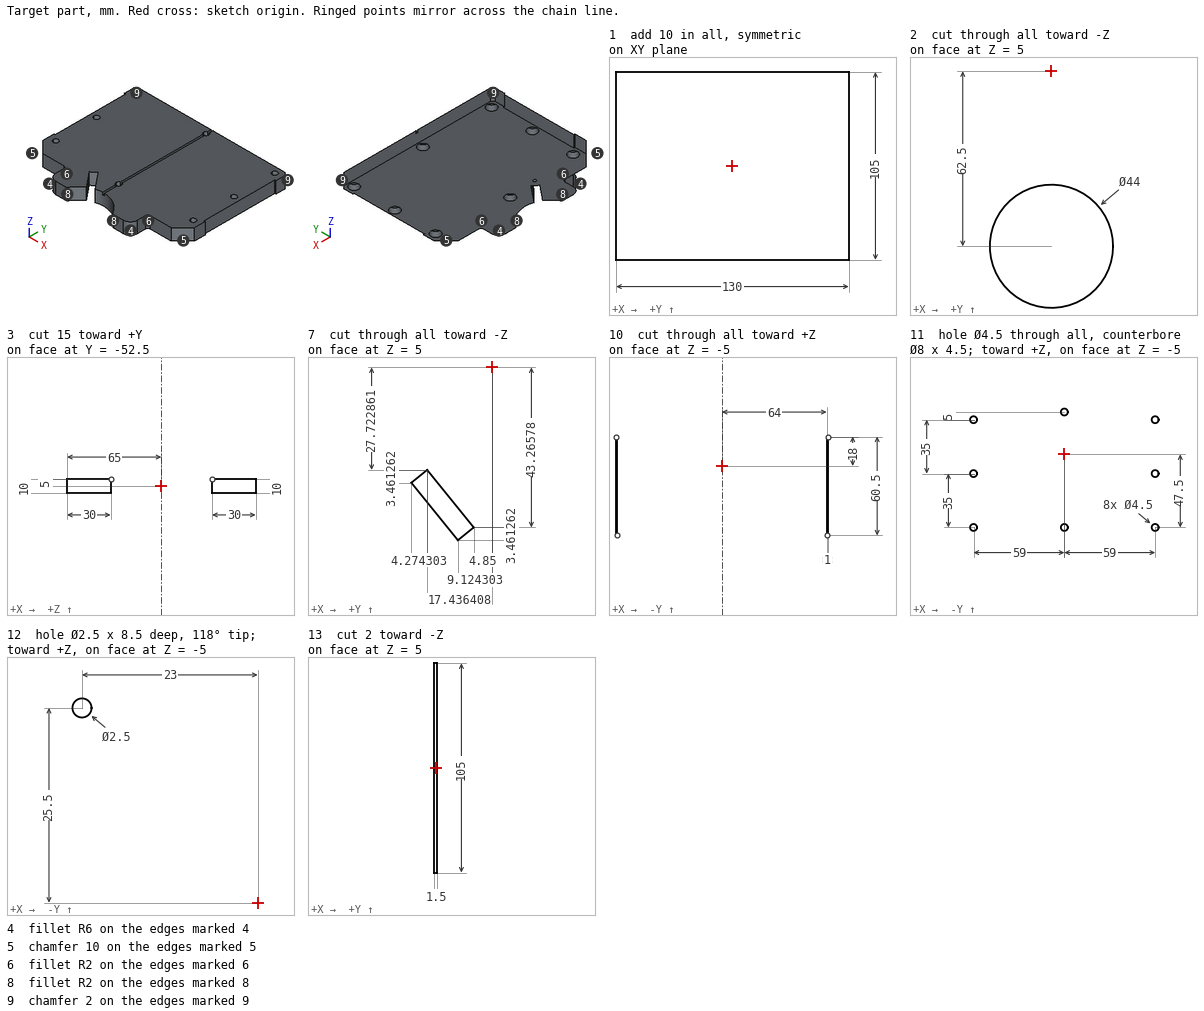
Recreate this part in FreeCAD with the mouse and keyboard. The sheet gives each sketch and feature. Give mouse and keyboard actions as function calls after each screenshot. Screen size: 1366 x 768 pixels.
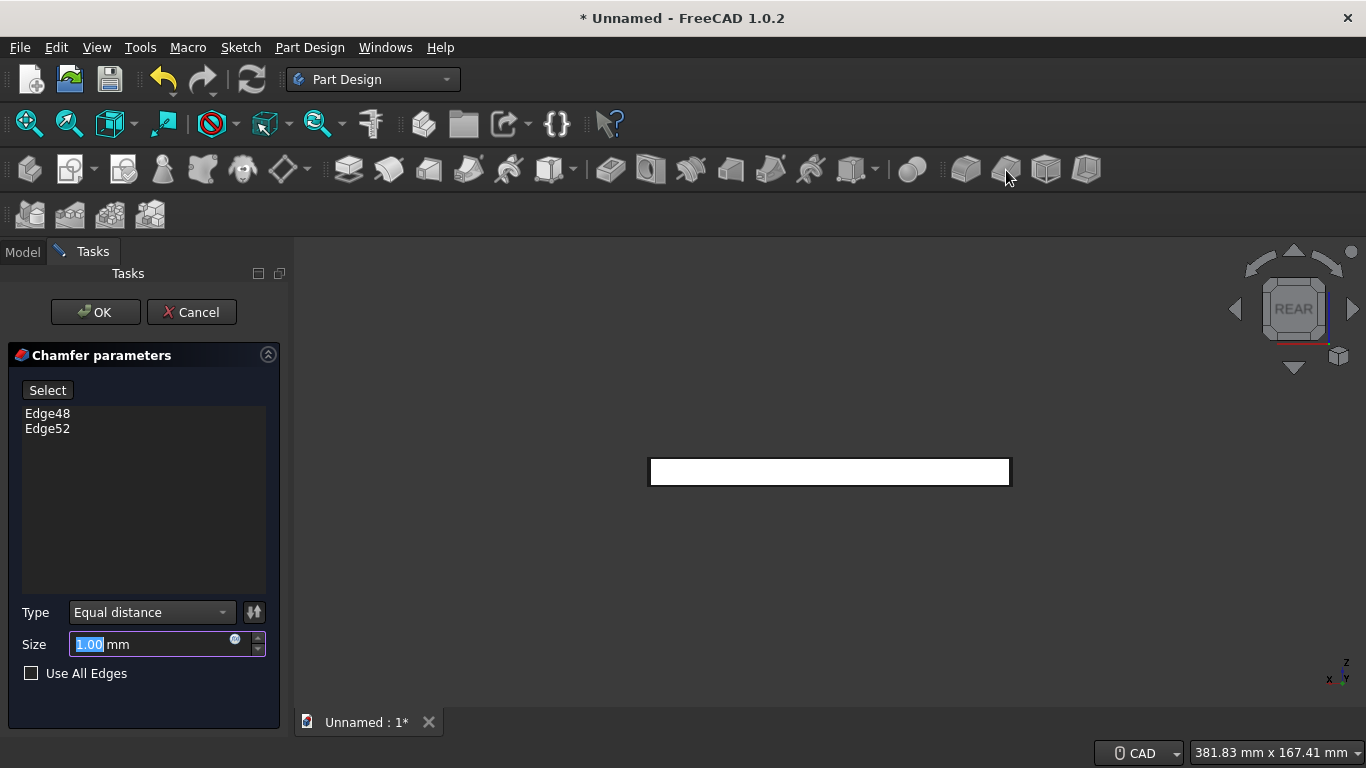
text(2)
key(Tab)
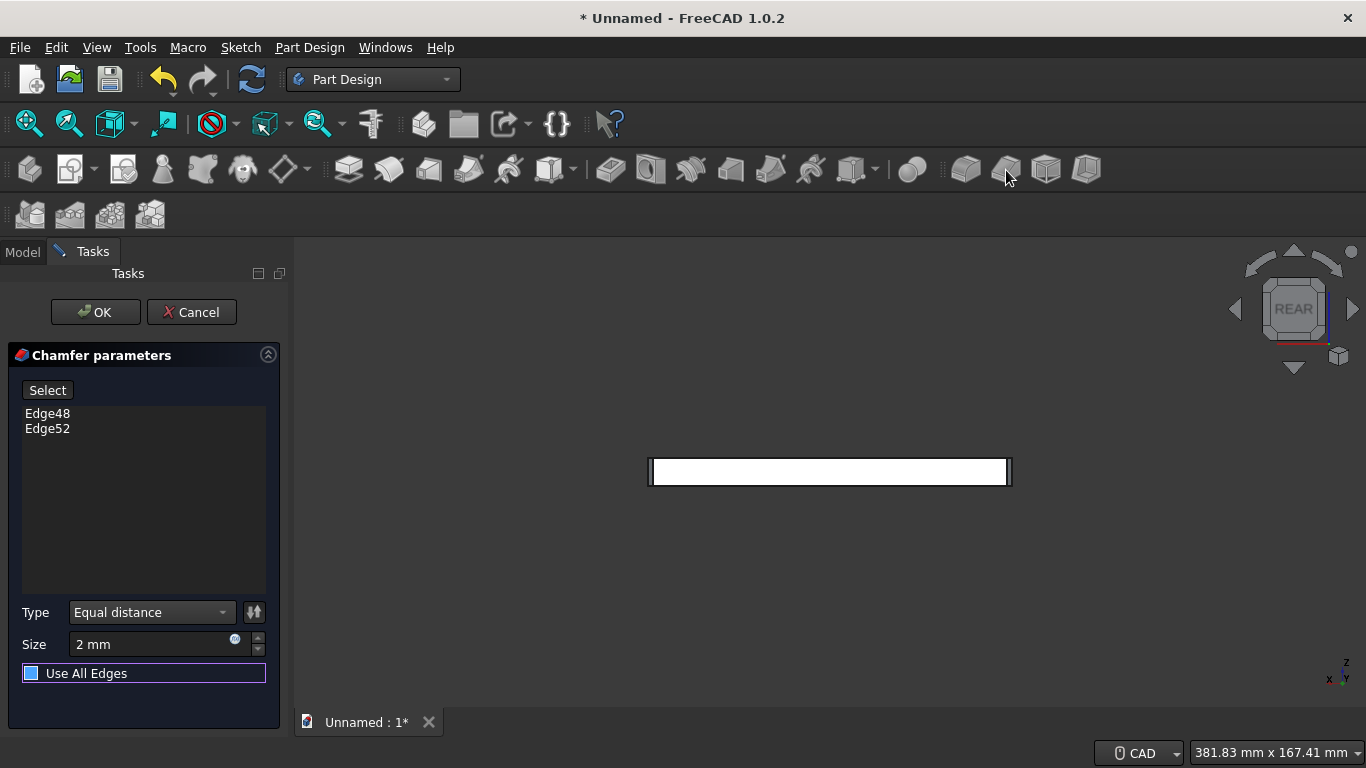
click(96, 312)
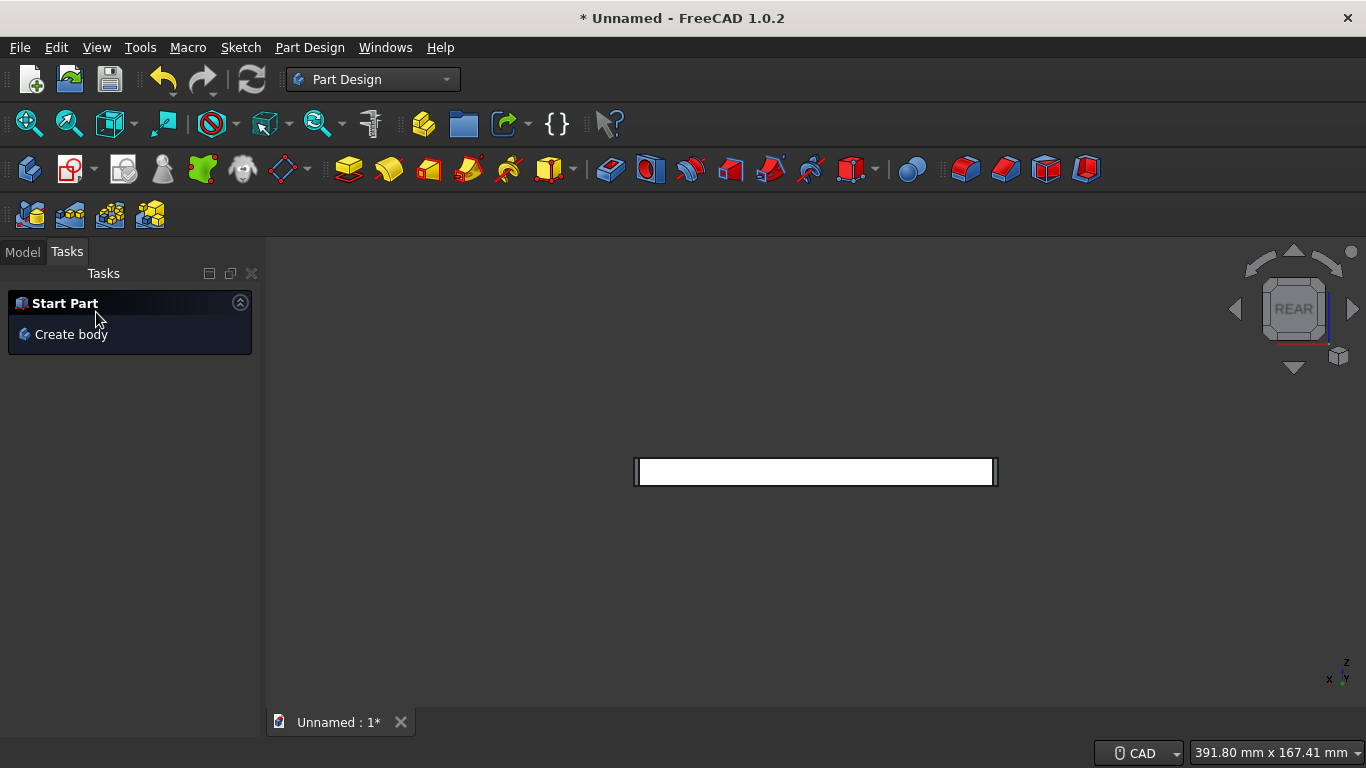
click(30, 124)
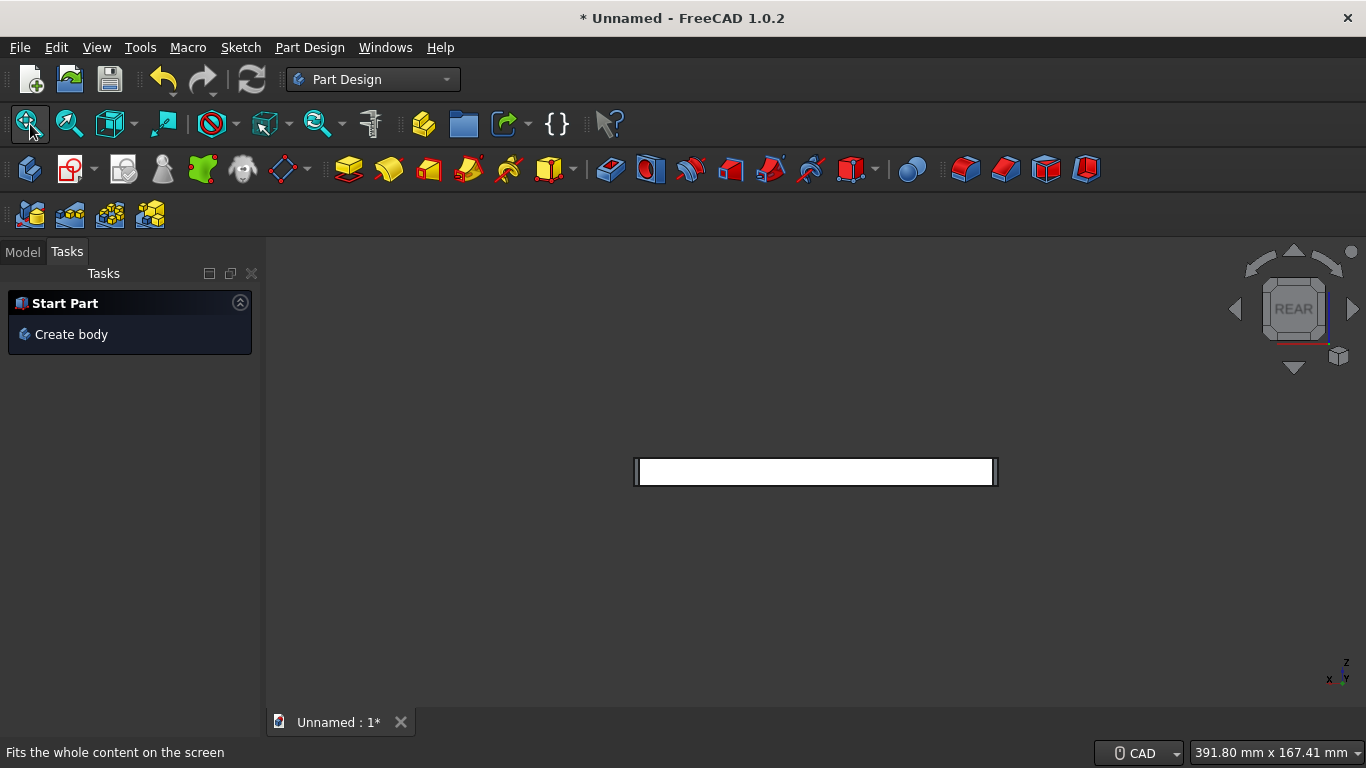
key(5)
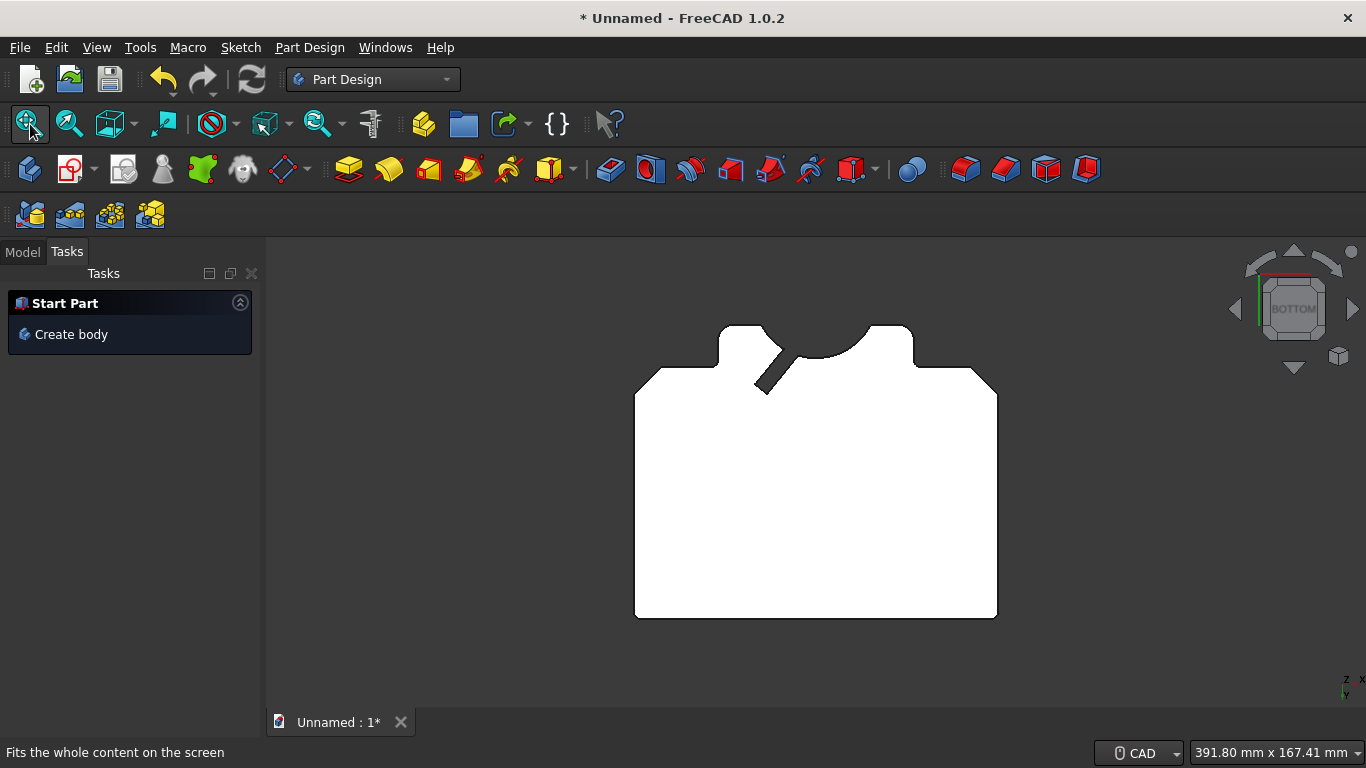
click(868, 471)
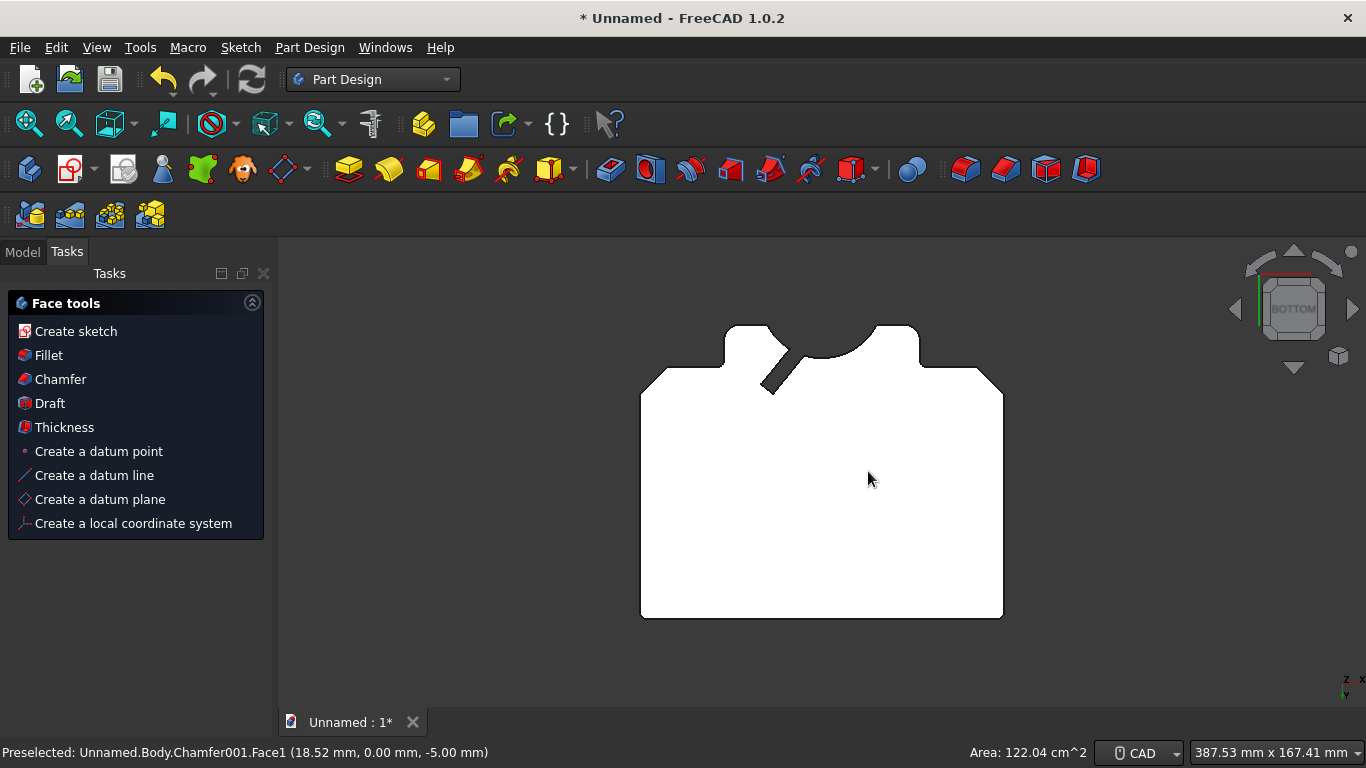
click(70, 170)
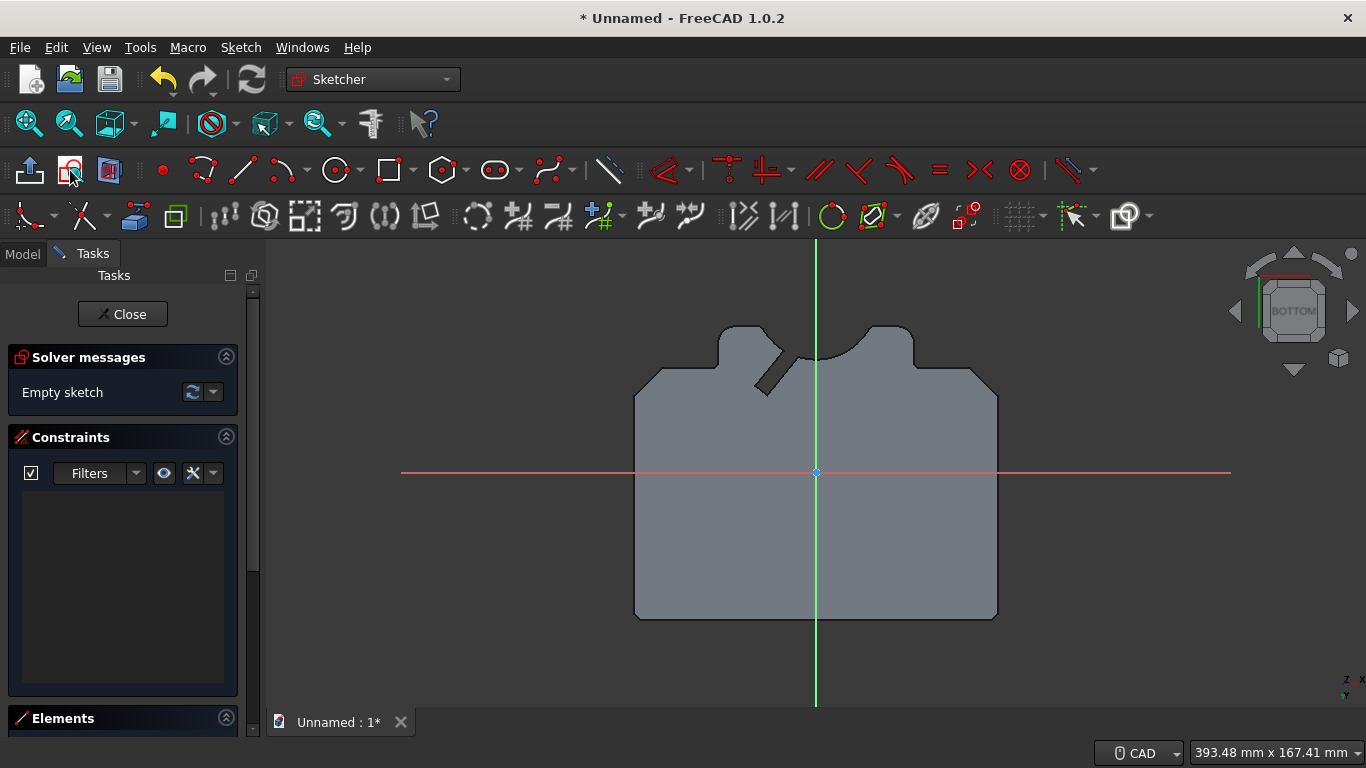
scroll(899, 549, up, 3)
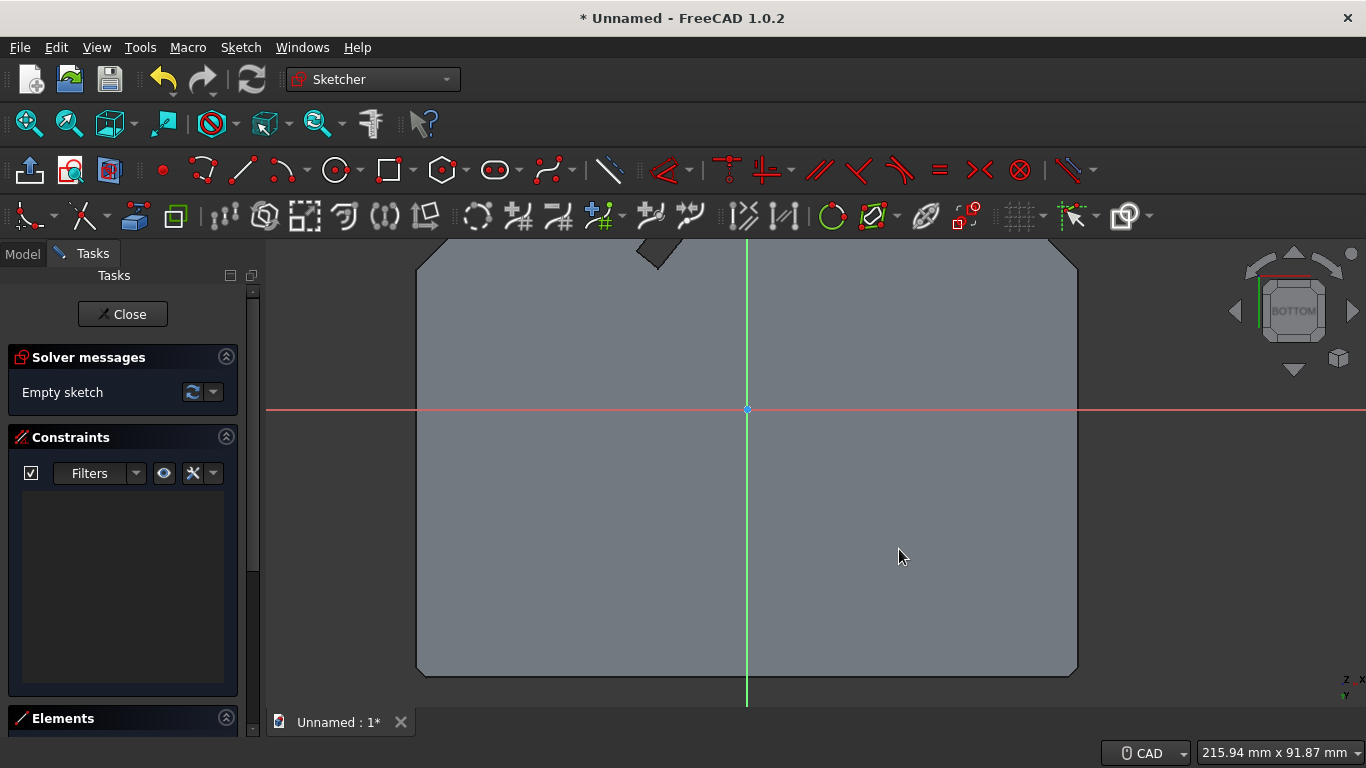
click(390, 170)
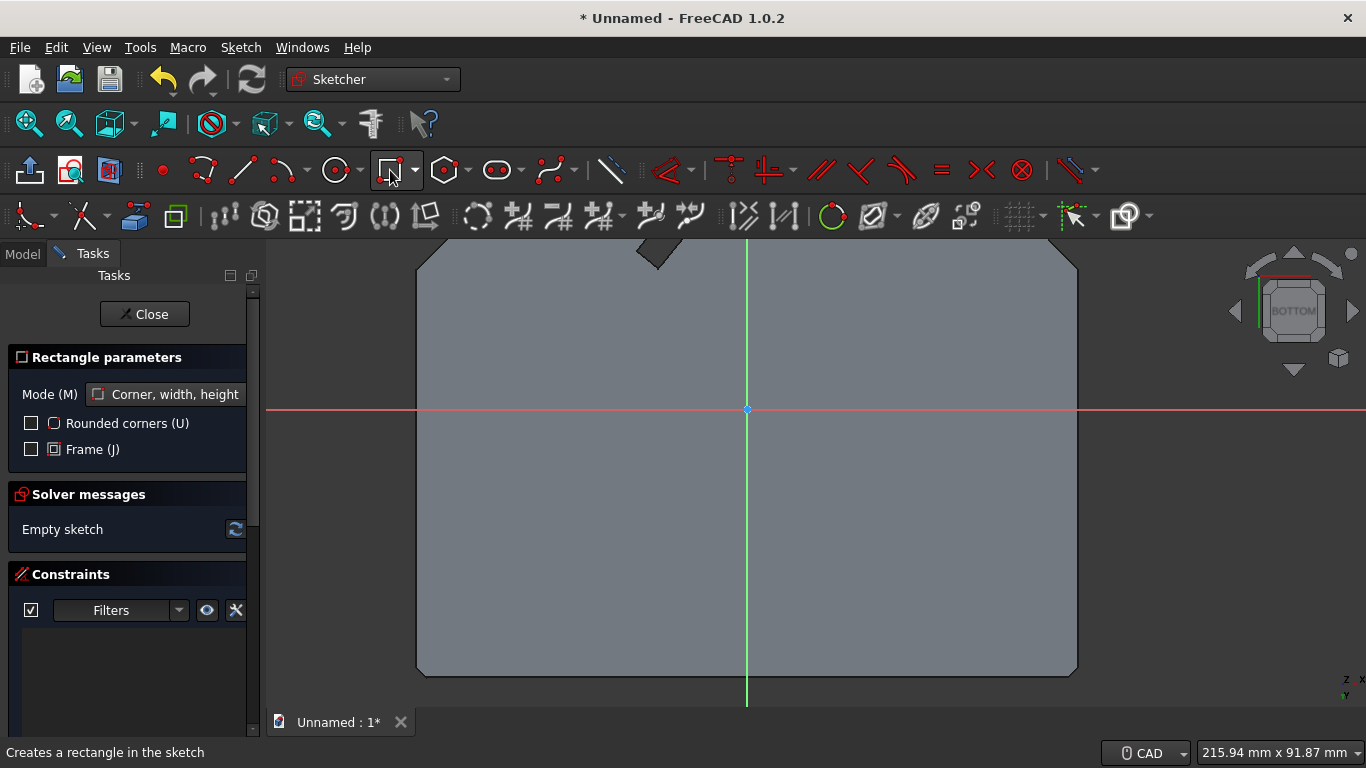
scroll(1073, 318, up, 6)